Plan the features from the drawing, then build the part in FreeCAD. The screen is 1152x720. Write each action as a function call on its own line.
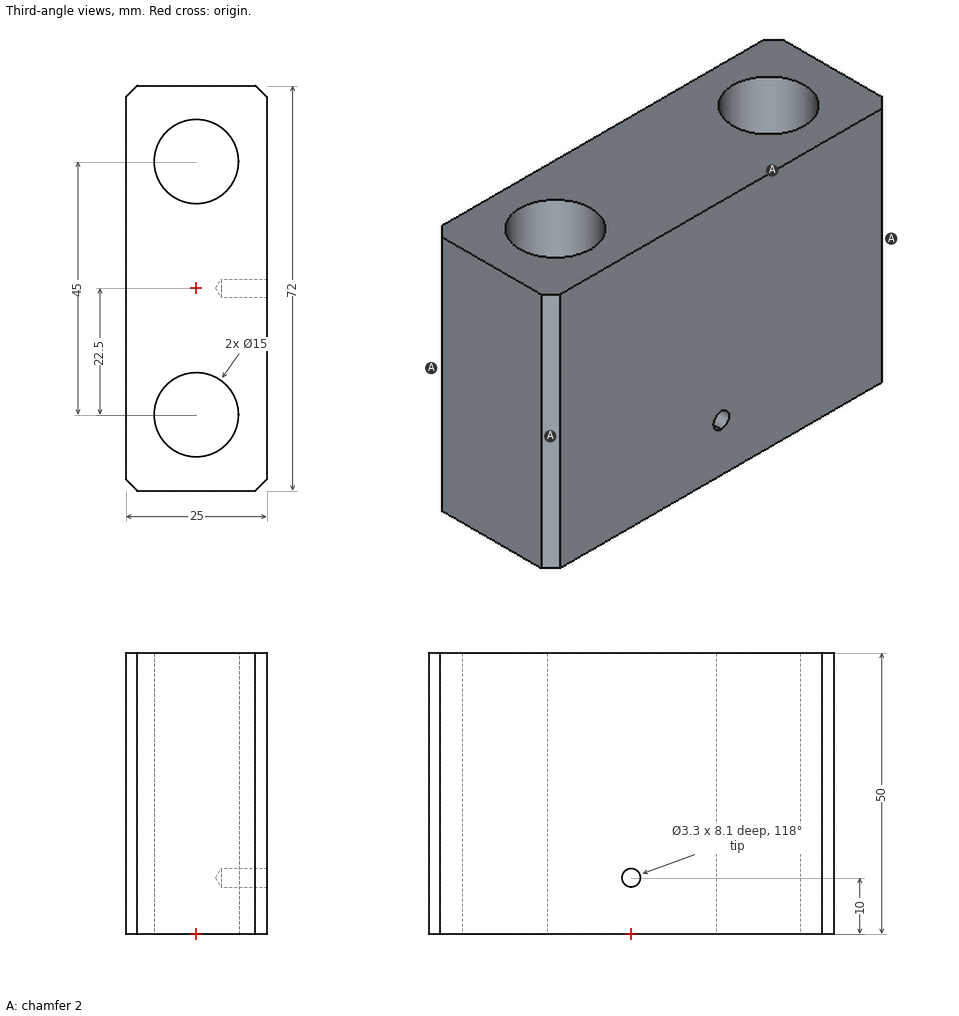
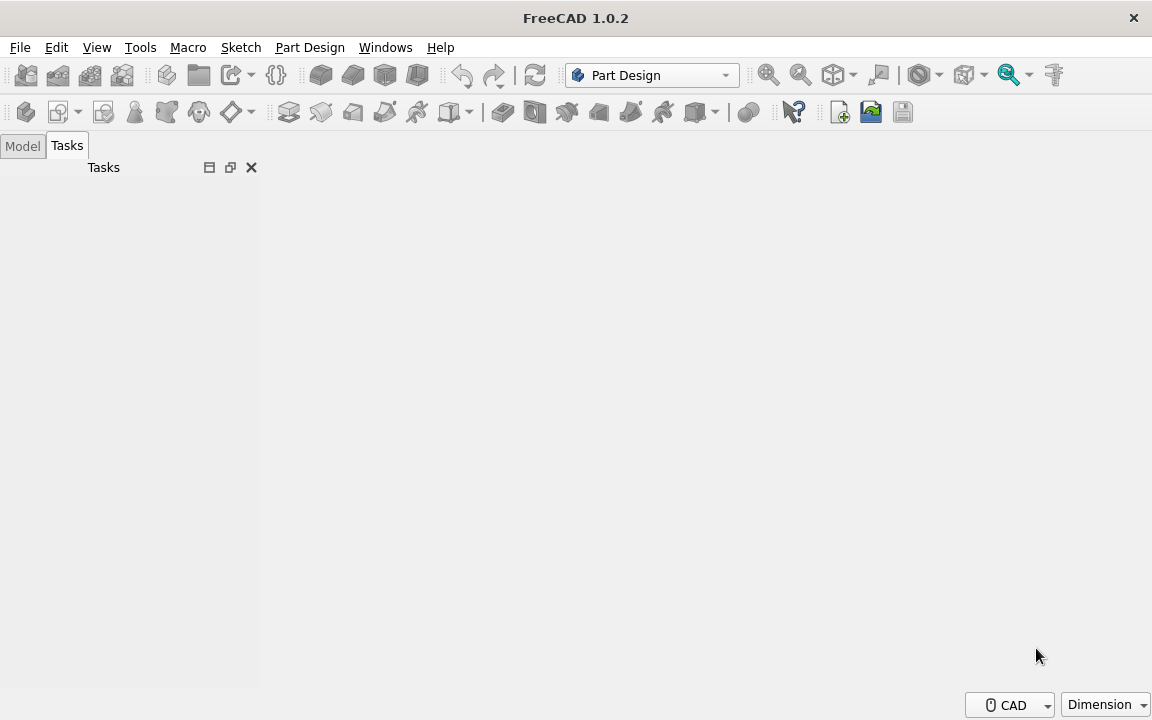
key(ctrl+n)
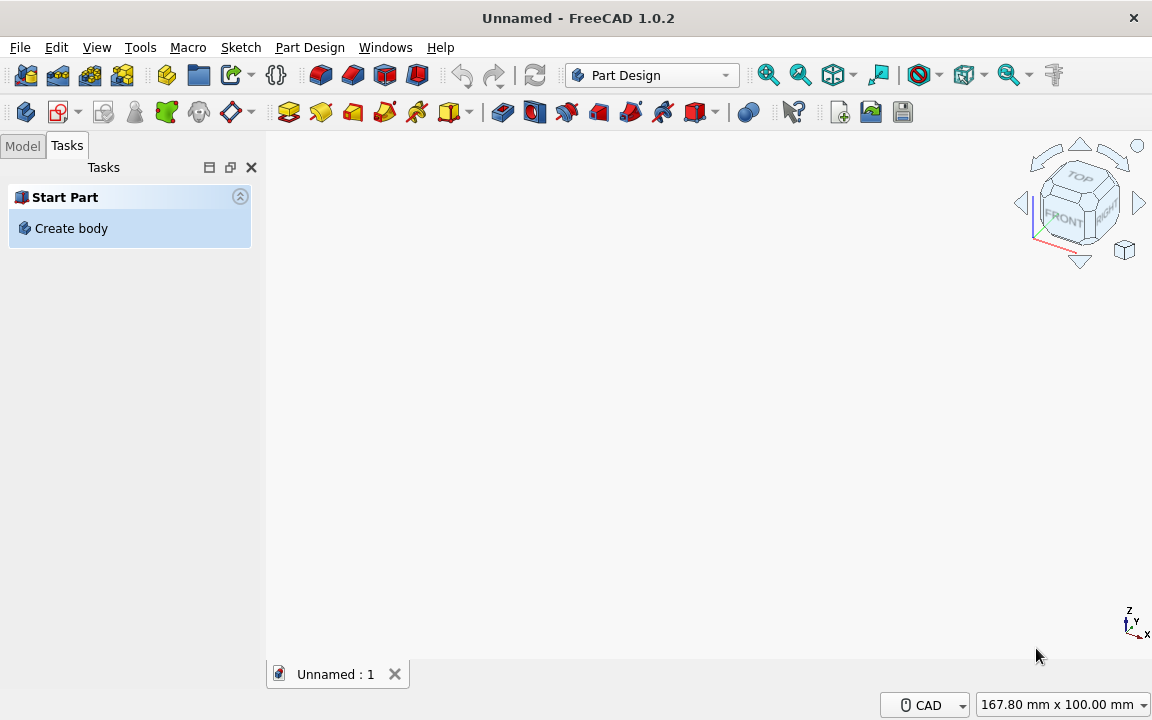
click(58, 112)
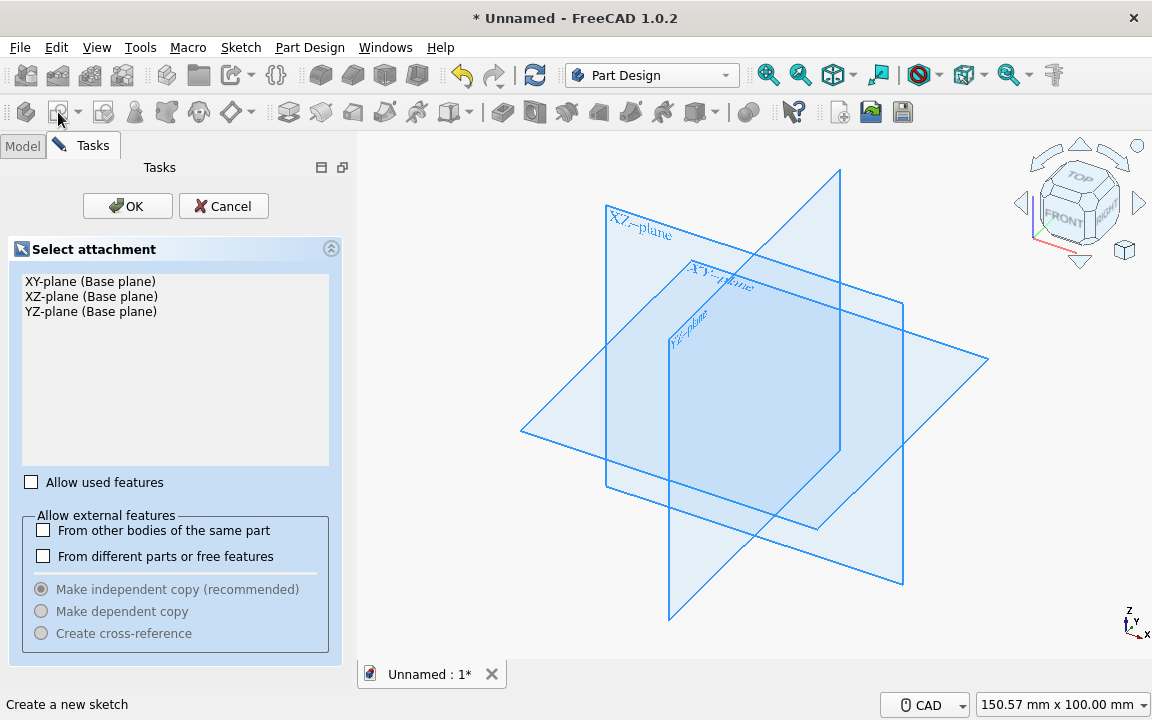
click(82, 282)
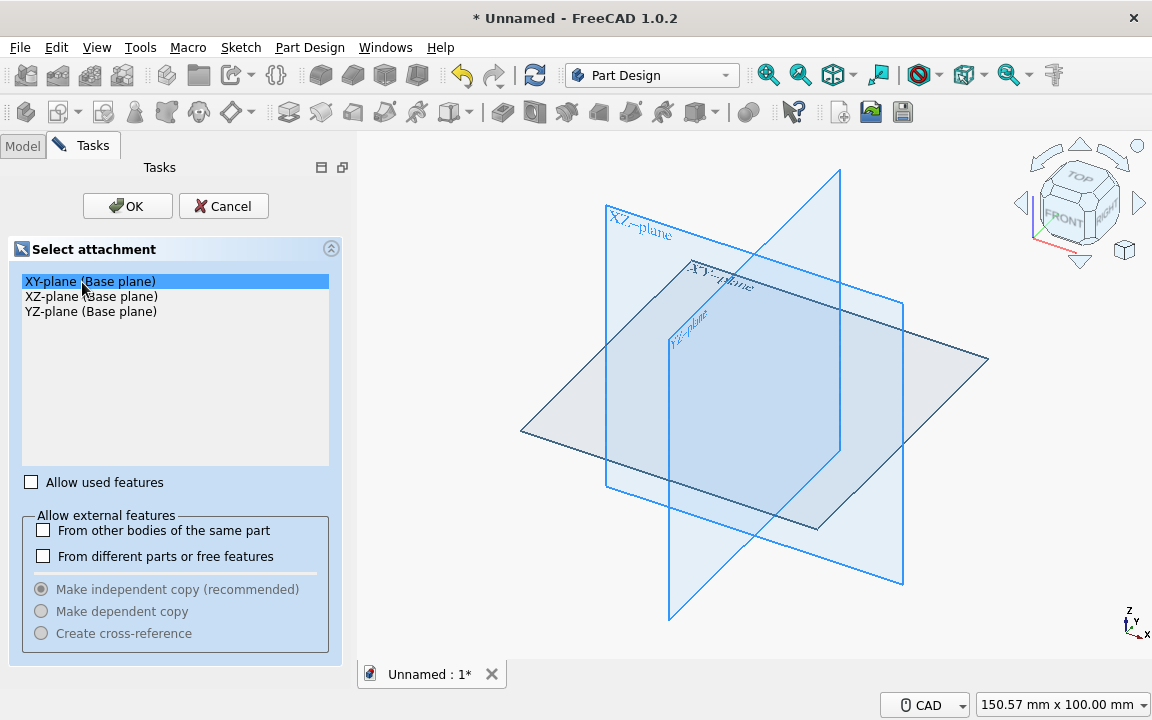
click(128, 206)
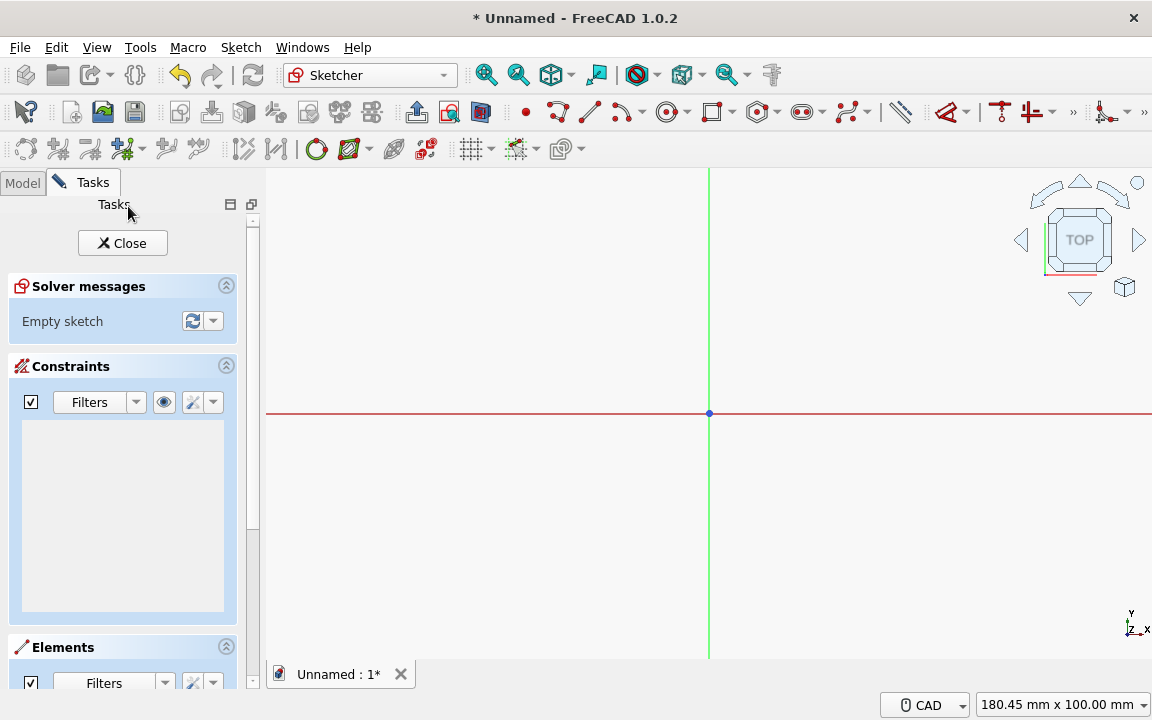
key(g)
key(v)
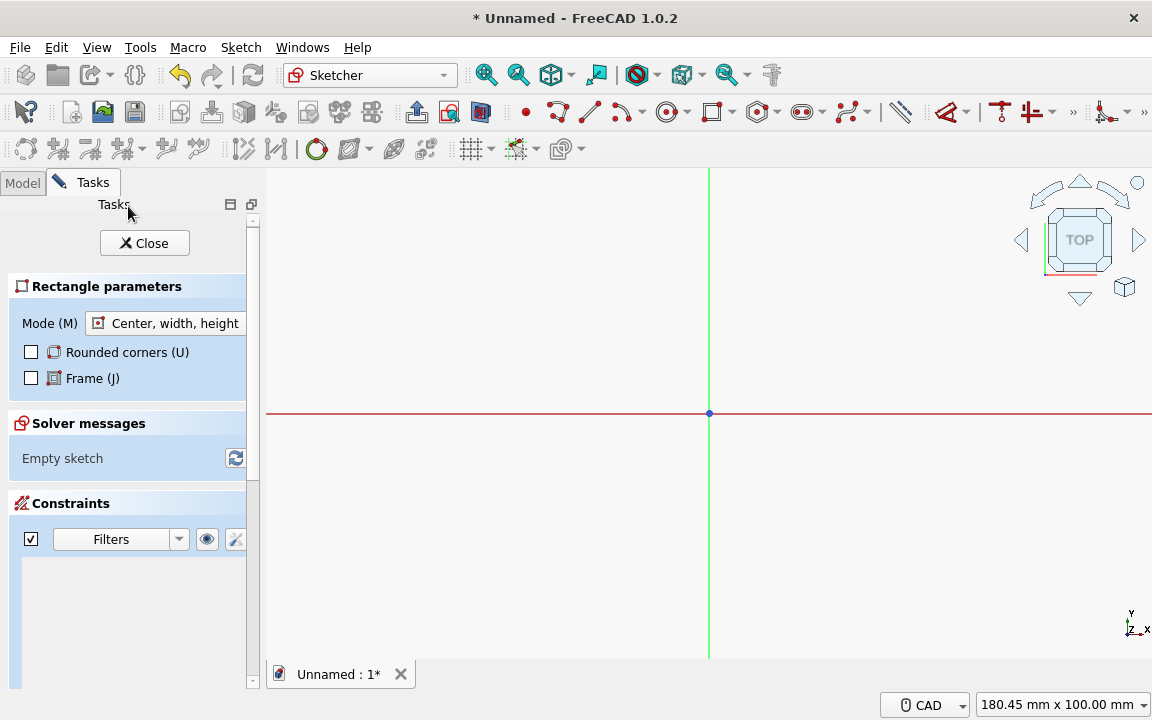
click(709, 414)
move(770, 237)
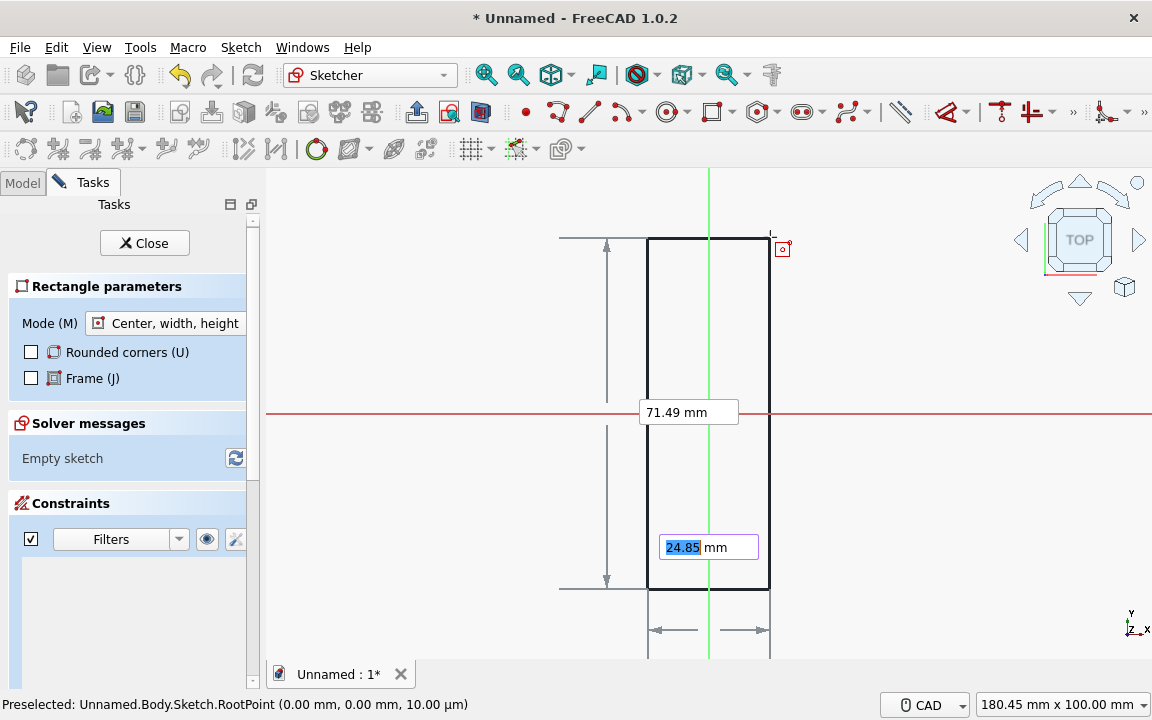
text(25)
key(Tab)
text(72)
key(Return)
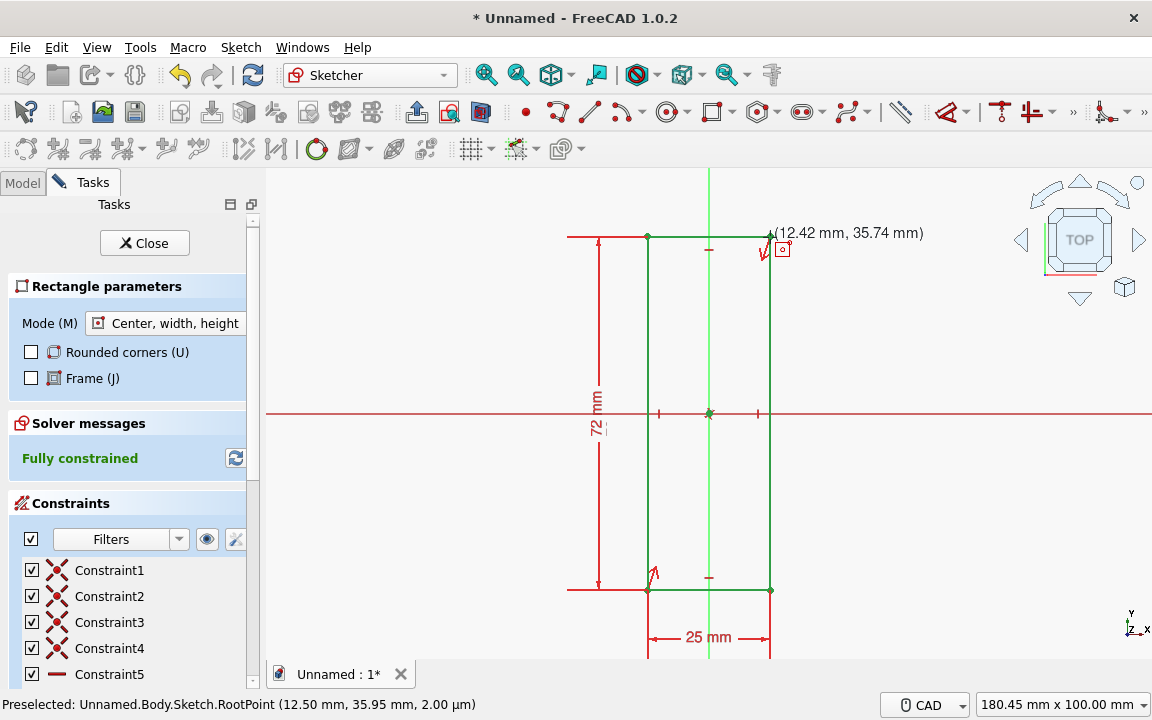
click(668, 112)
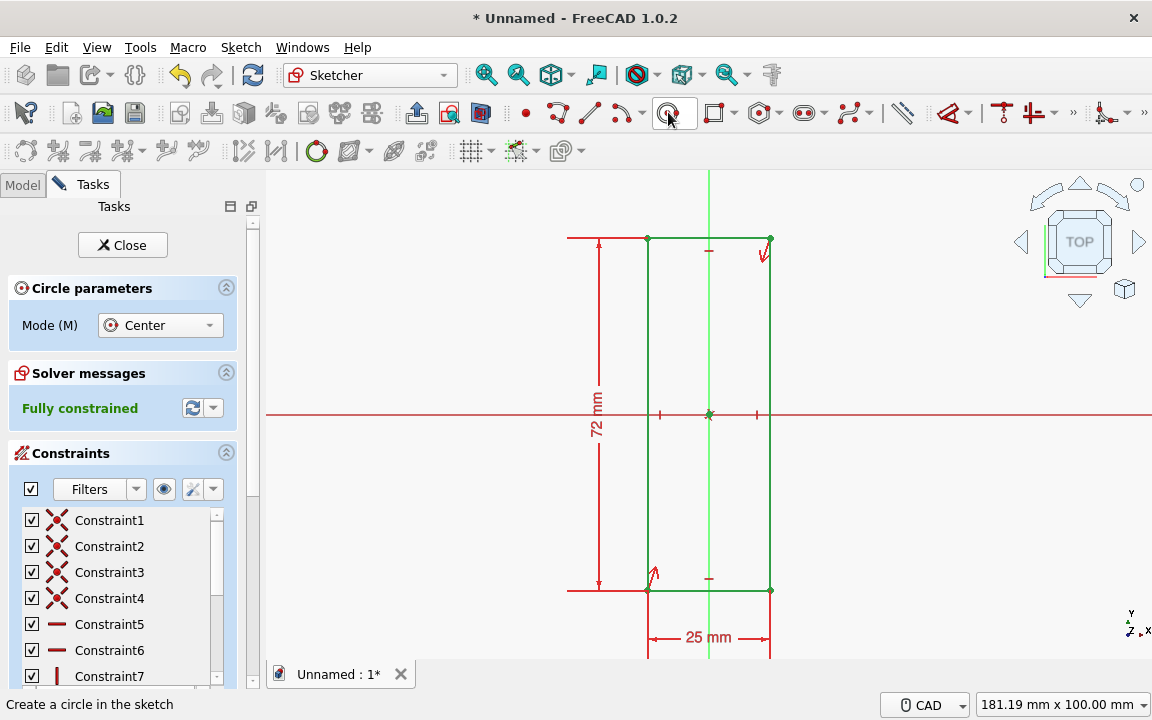
click(709, 525)
move(735, 499)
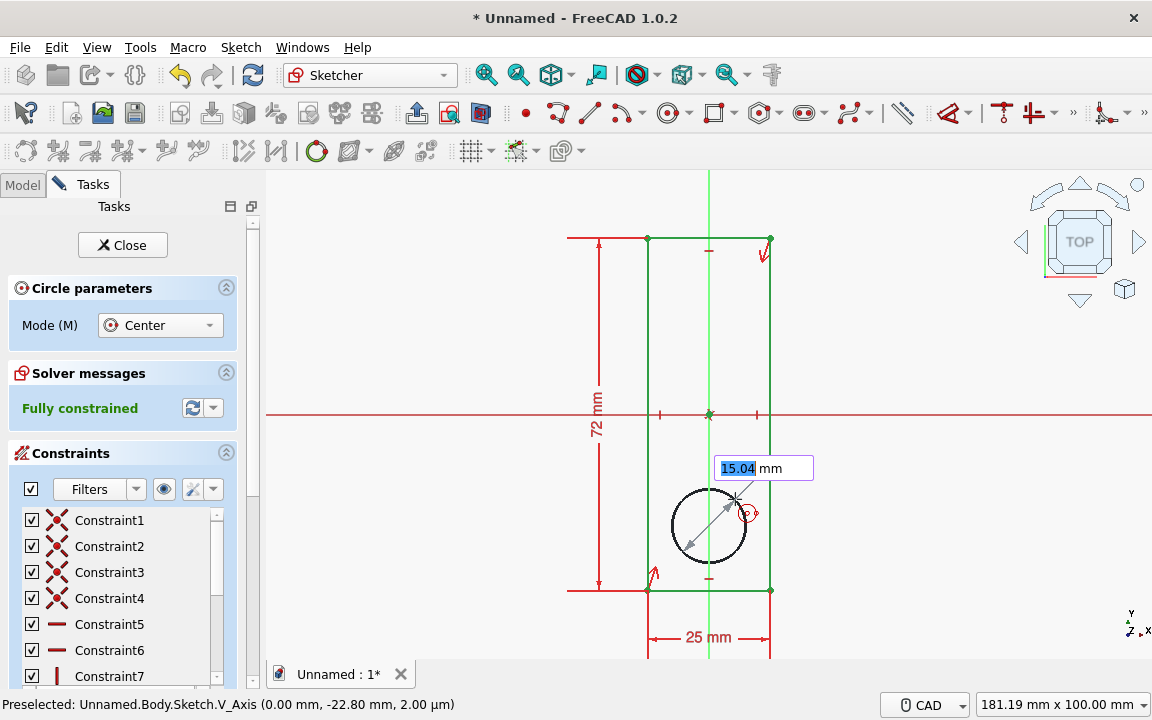
text(15)
key(Return)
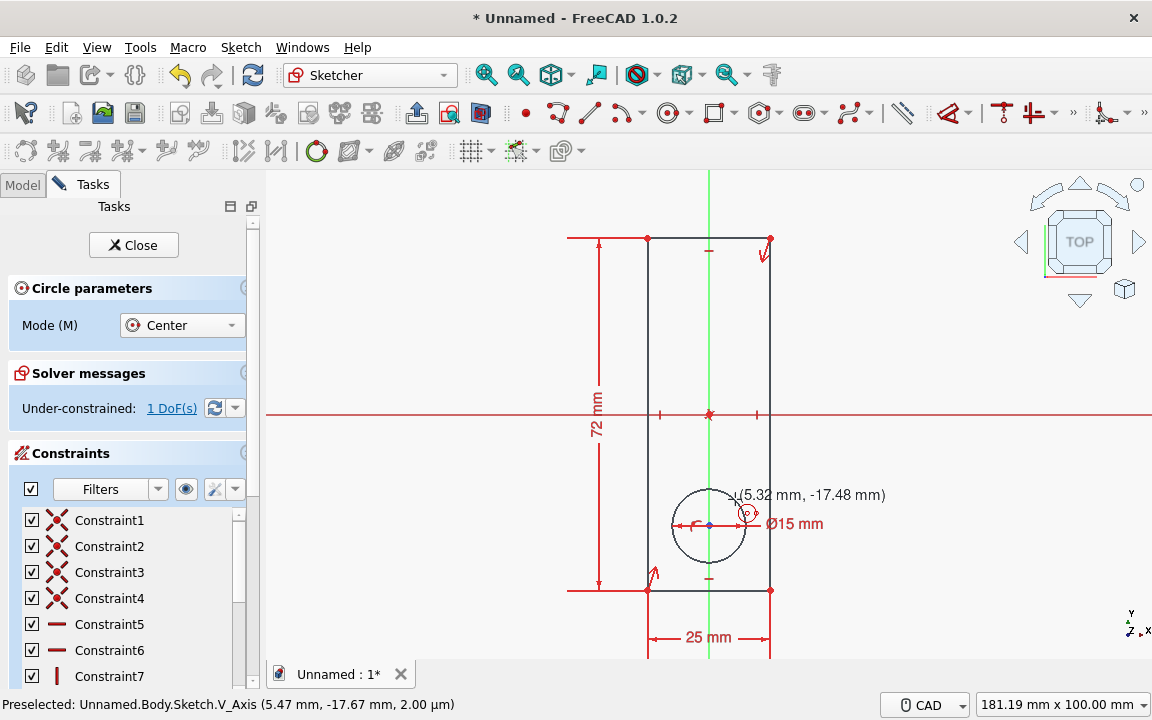
click(709, 304)
move(735, 279)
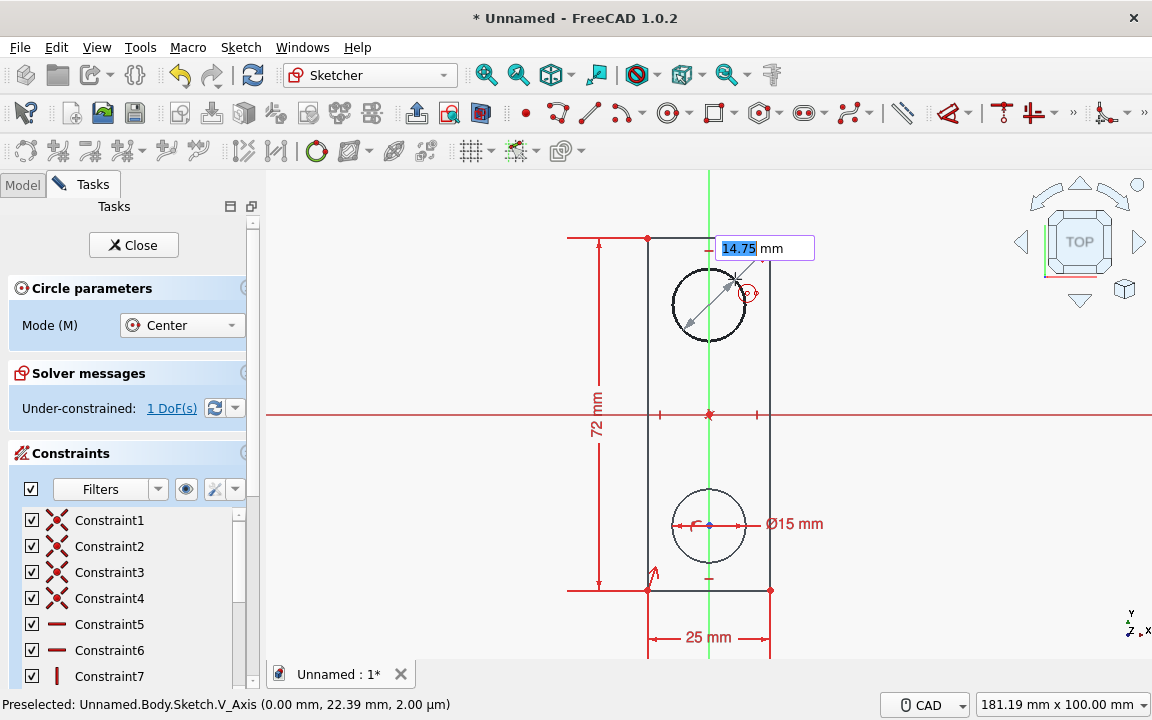
text(15)
key(Return)
key(Escape)